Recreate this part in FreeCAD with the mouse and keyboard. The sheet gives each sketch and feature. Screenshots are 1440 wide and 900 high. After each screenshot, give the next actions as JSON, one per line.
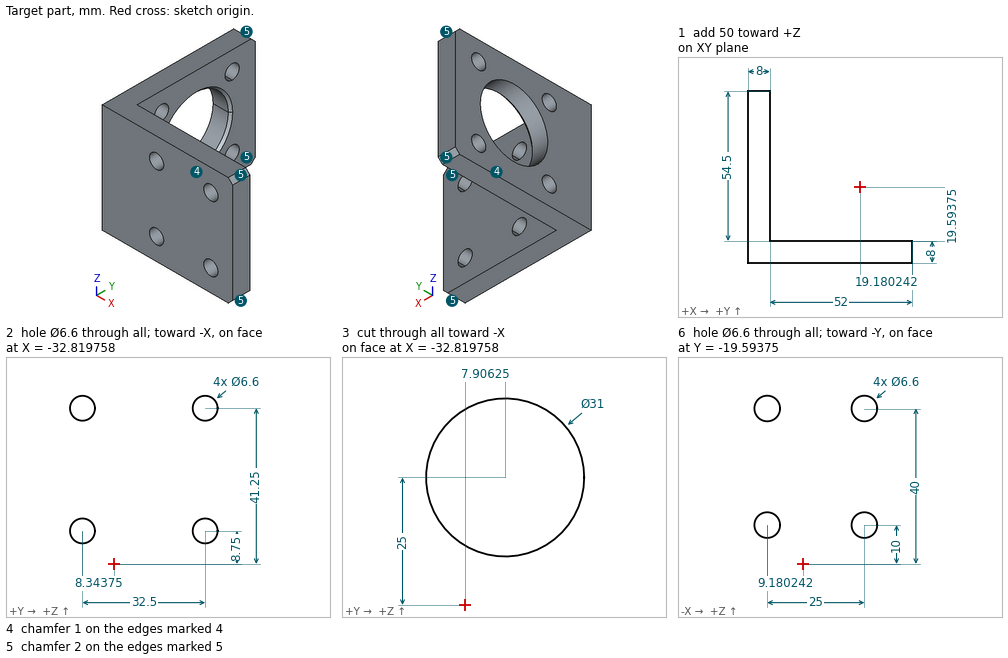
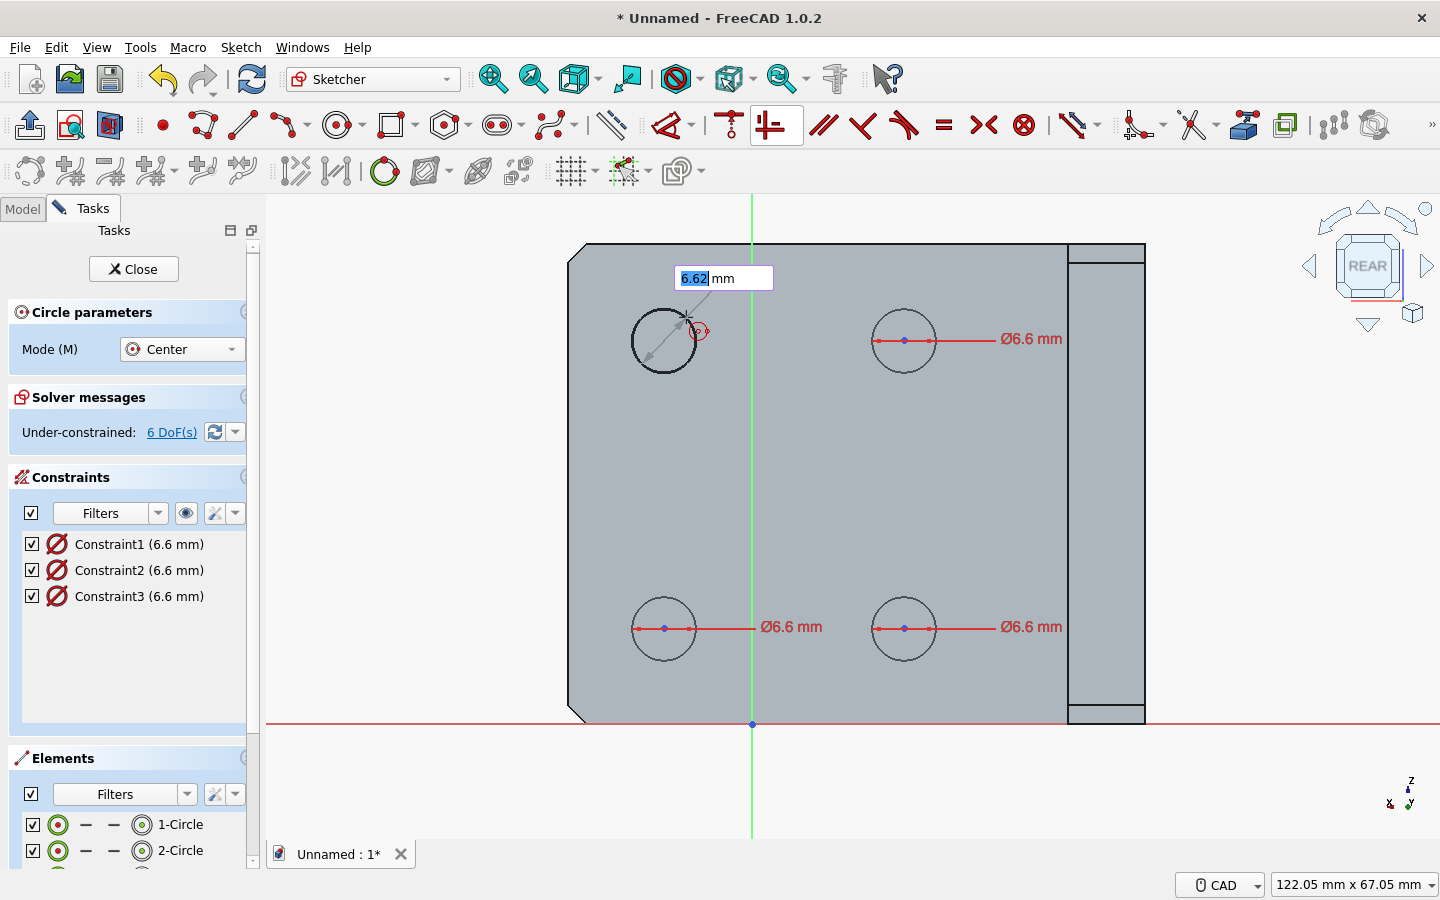
{"action": "type", "text": "6.6"}
{"action": "key", "text": "Return"}
{"action": "key", "text": "Escape"}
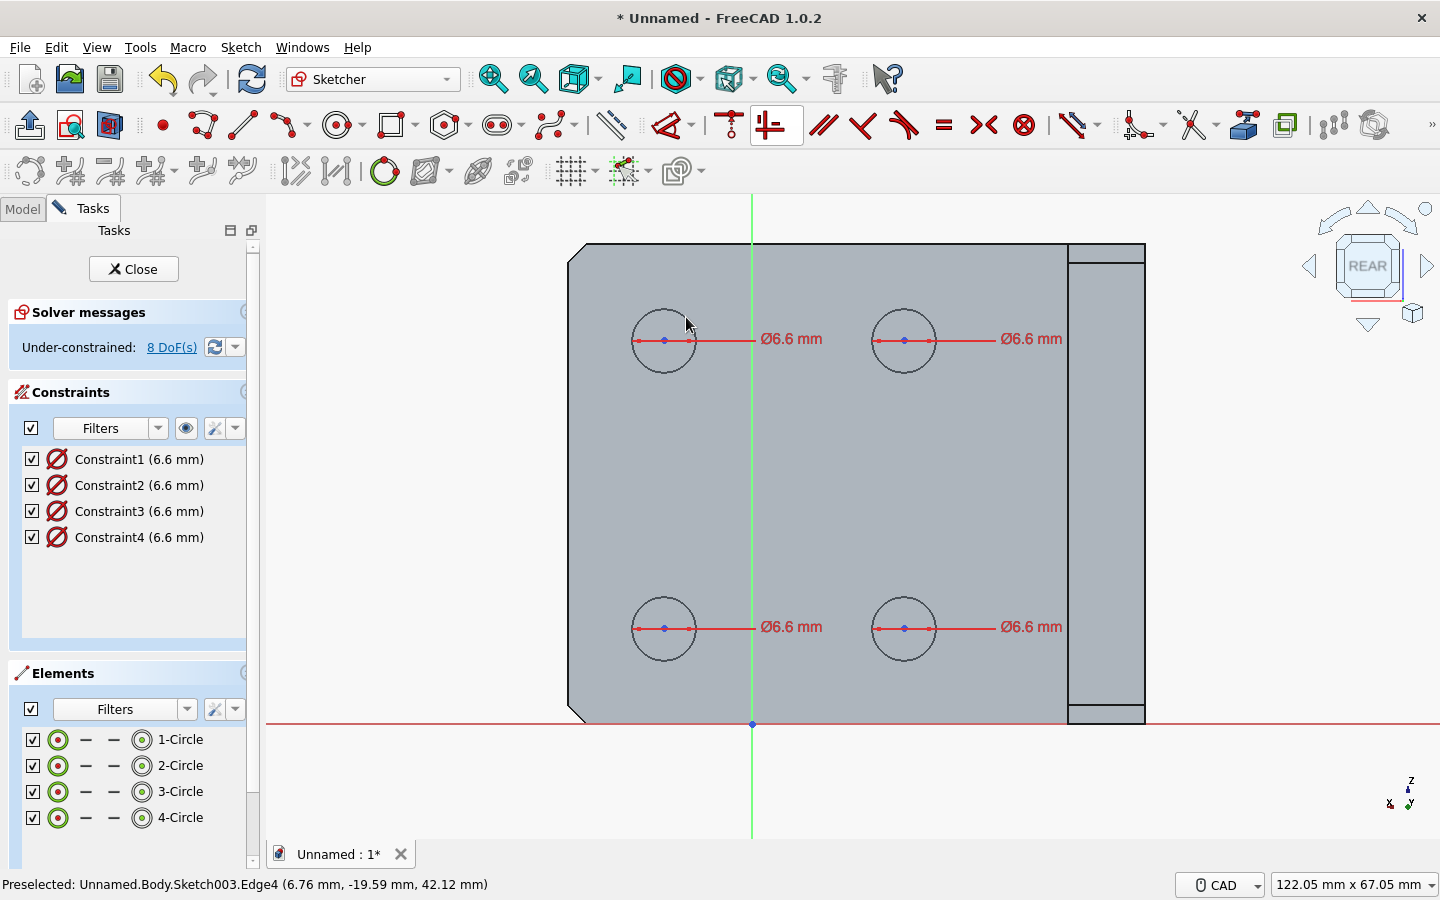
{"action": "left_click", "coordinate": [904, 341]}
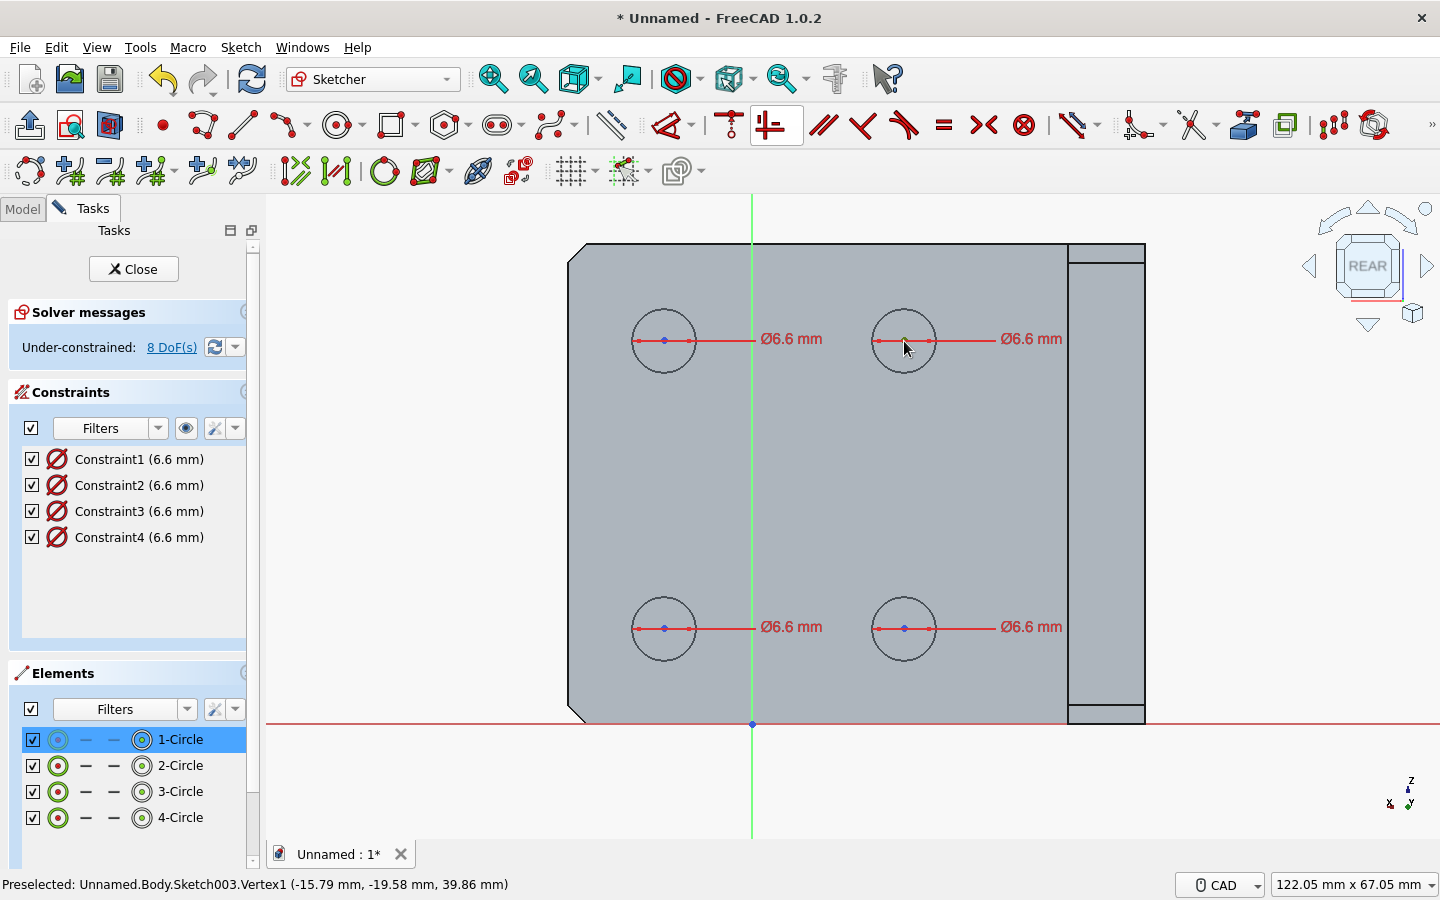
{"action": "left_click", "coordinate": [904, 629]}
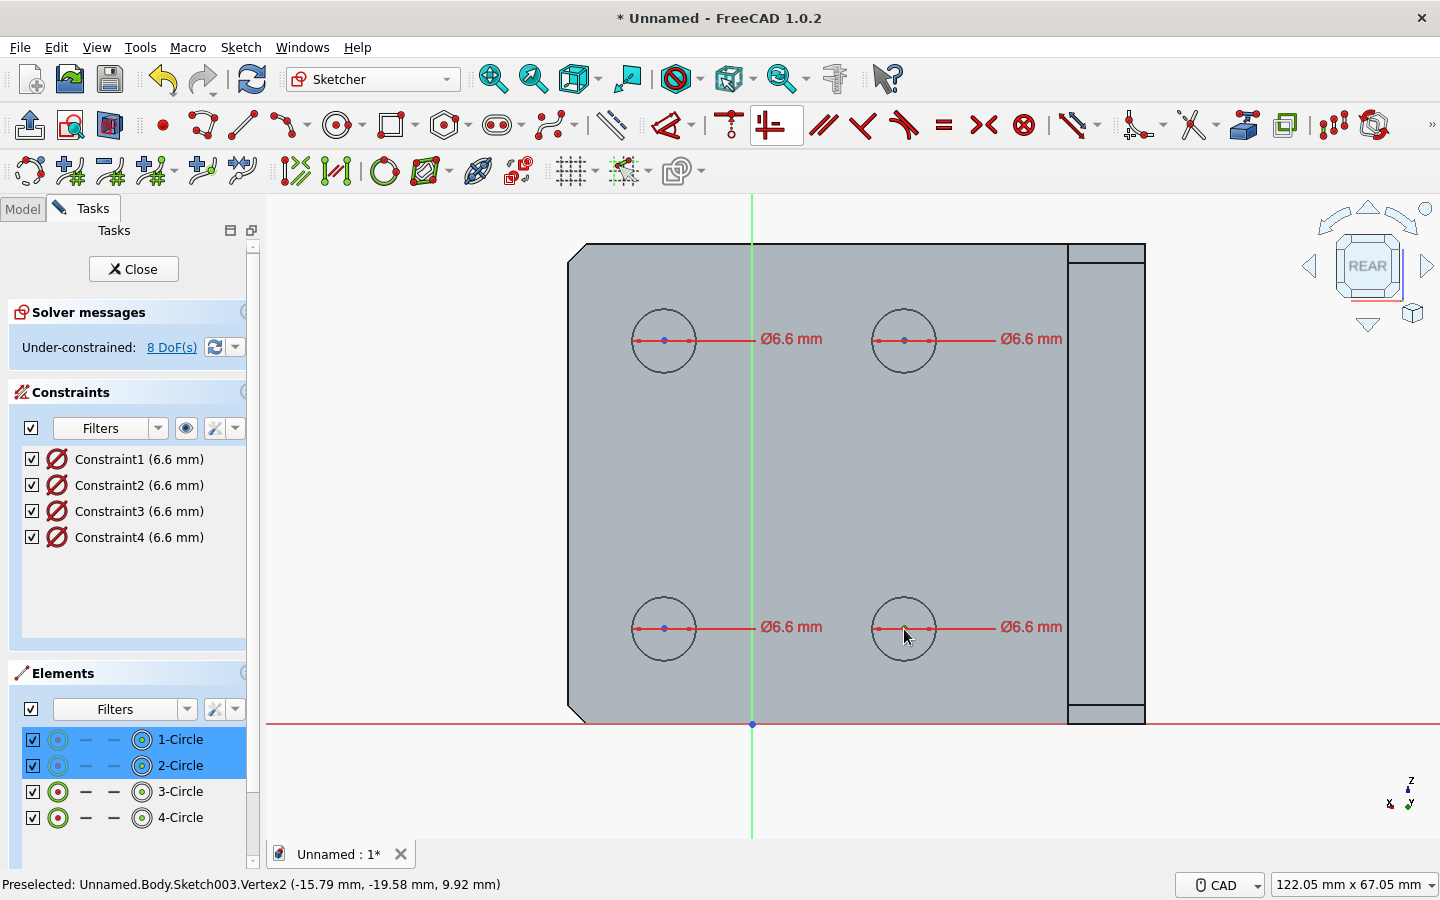
{"action": "key", "text": "v"}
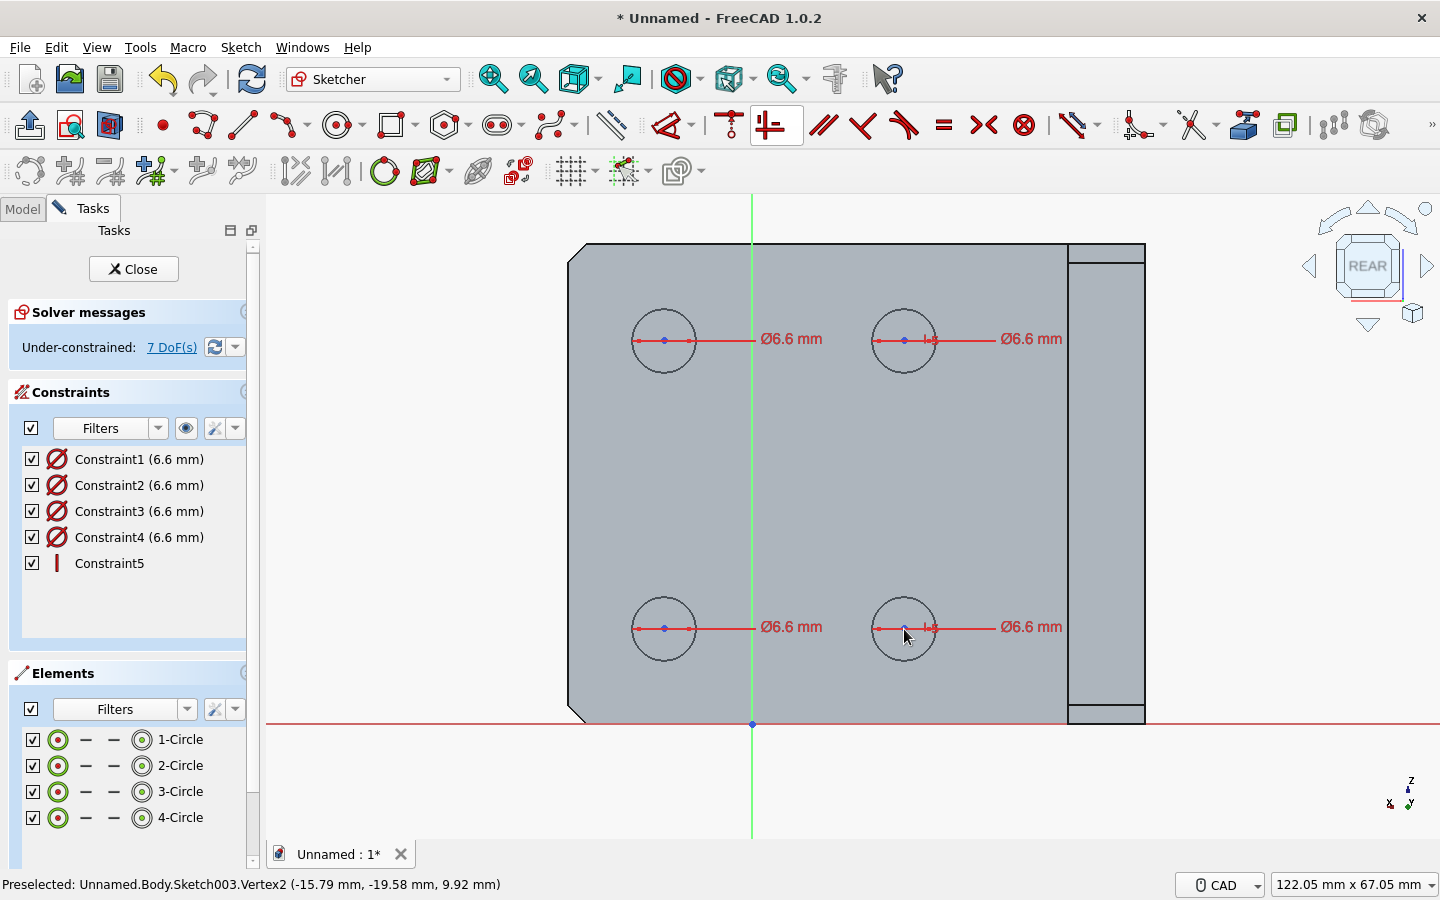
{"action": "left_click", "coordinate": [904, 629]}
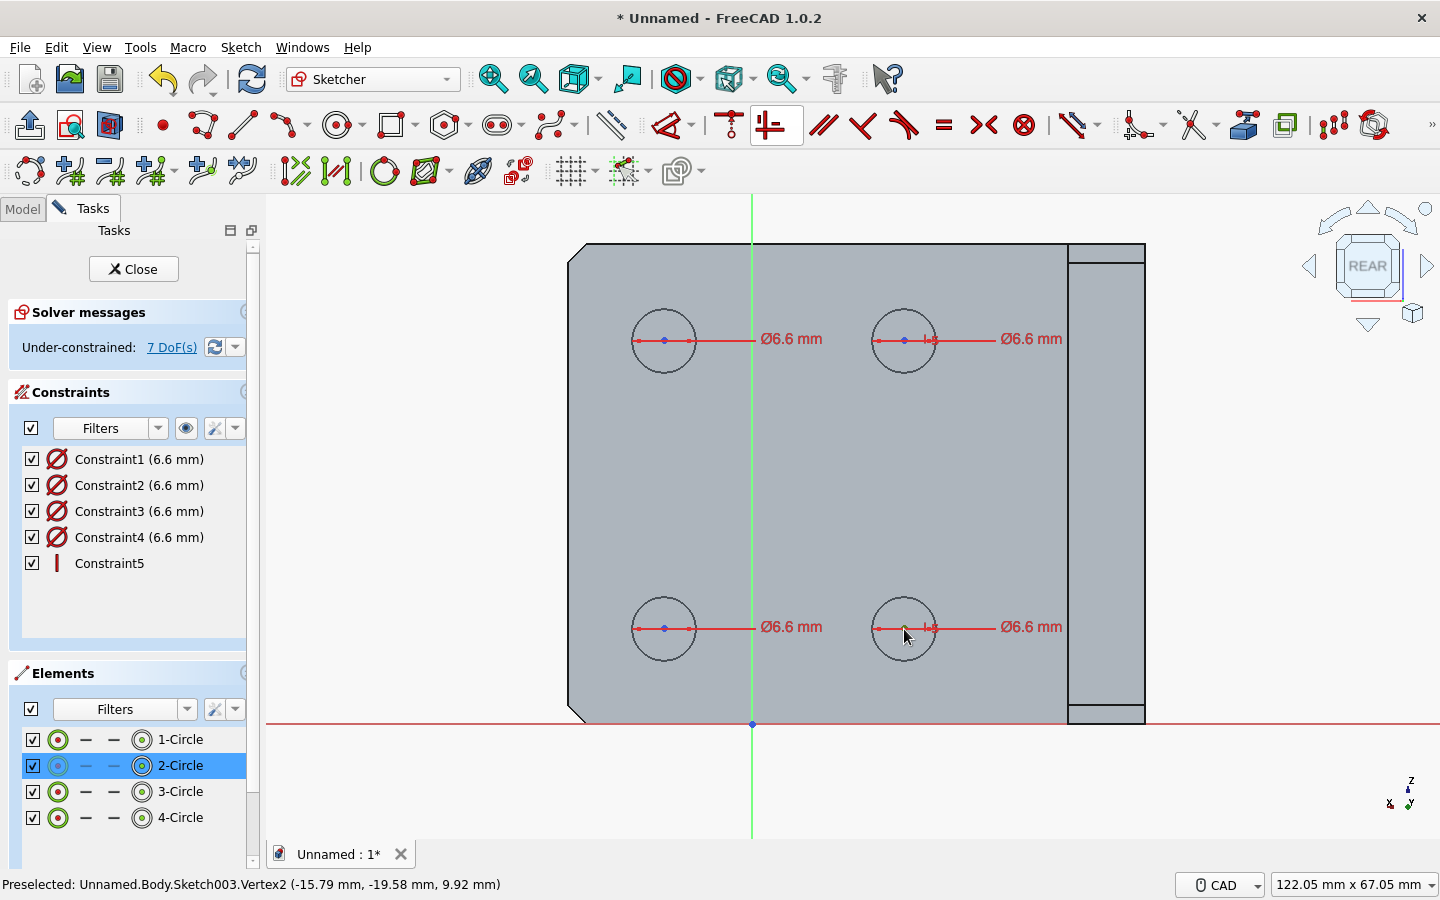
{"action": "left_click", "coordinate": [664, 629]}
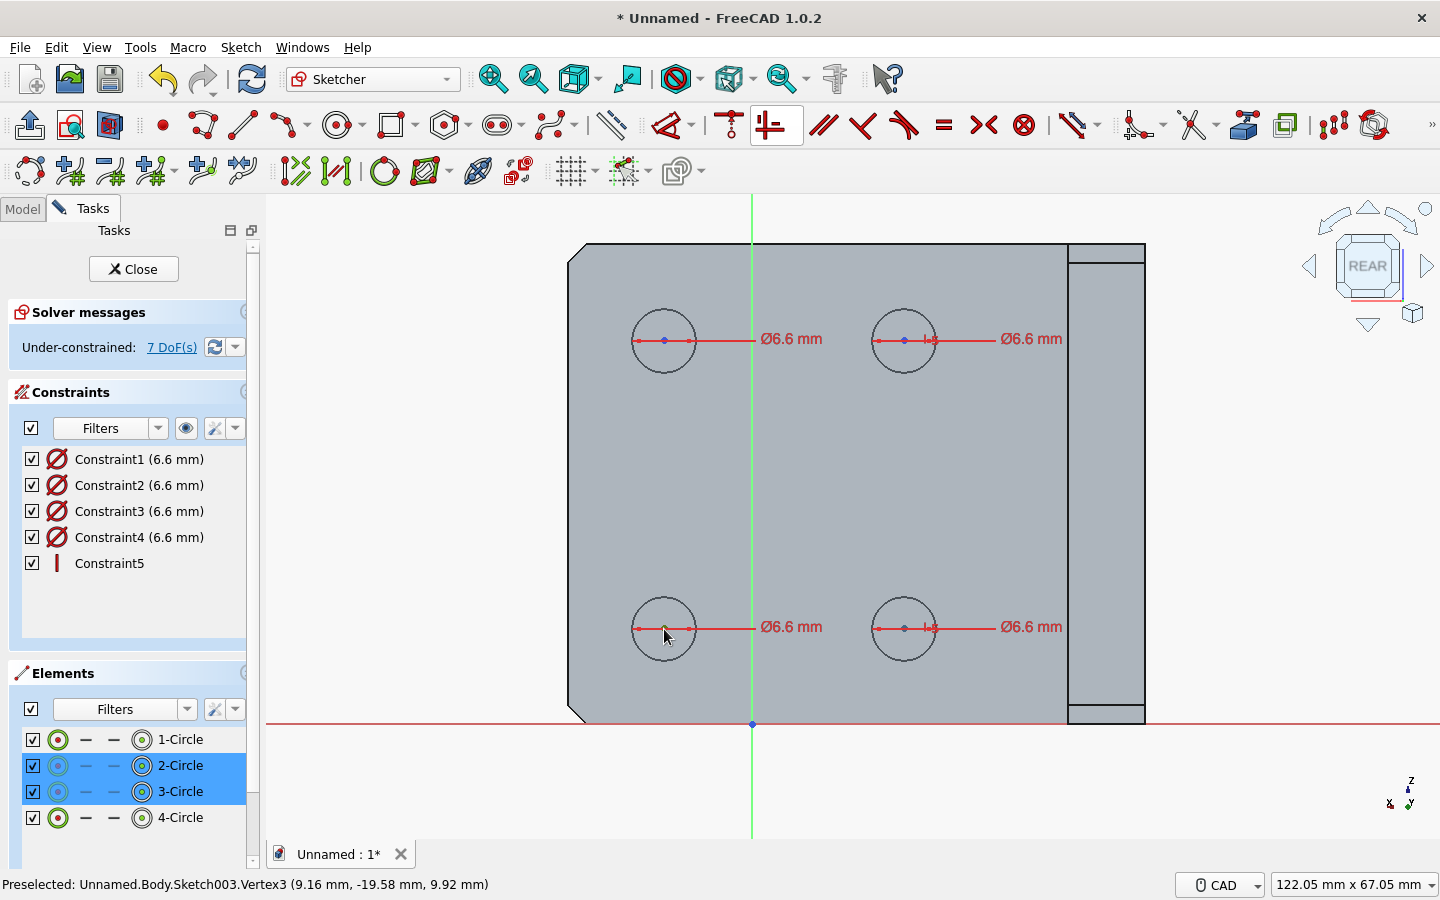
{"action": "key", "text": "h"}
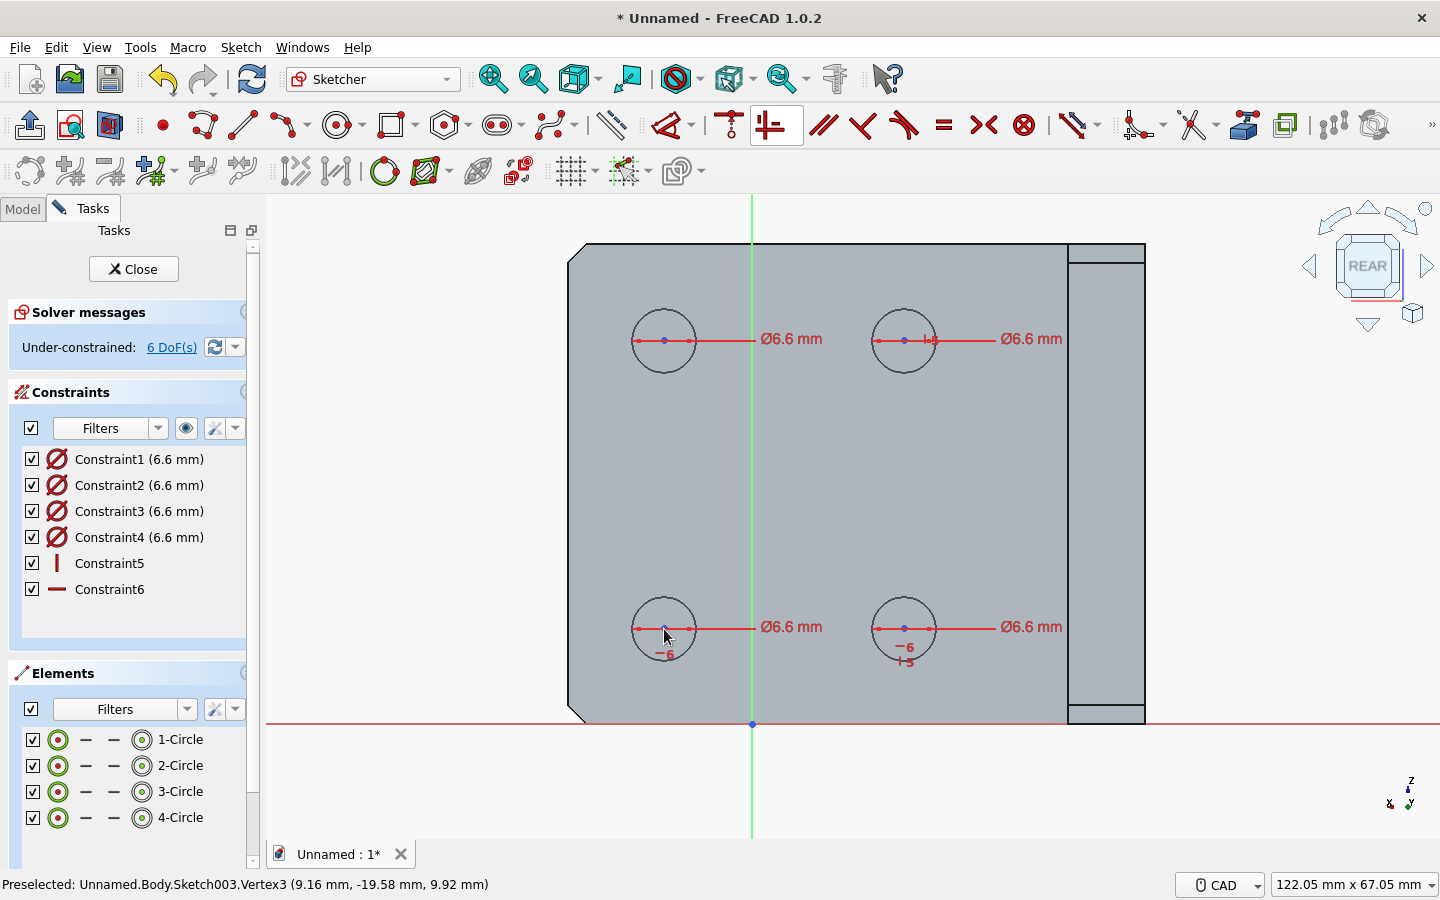
{"action": "left_click", "coordinate": [664, 629]}